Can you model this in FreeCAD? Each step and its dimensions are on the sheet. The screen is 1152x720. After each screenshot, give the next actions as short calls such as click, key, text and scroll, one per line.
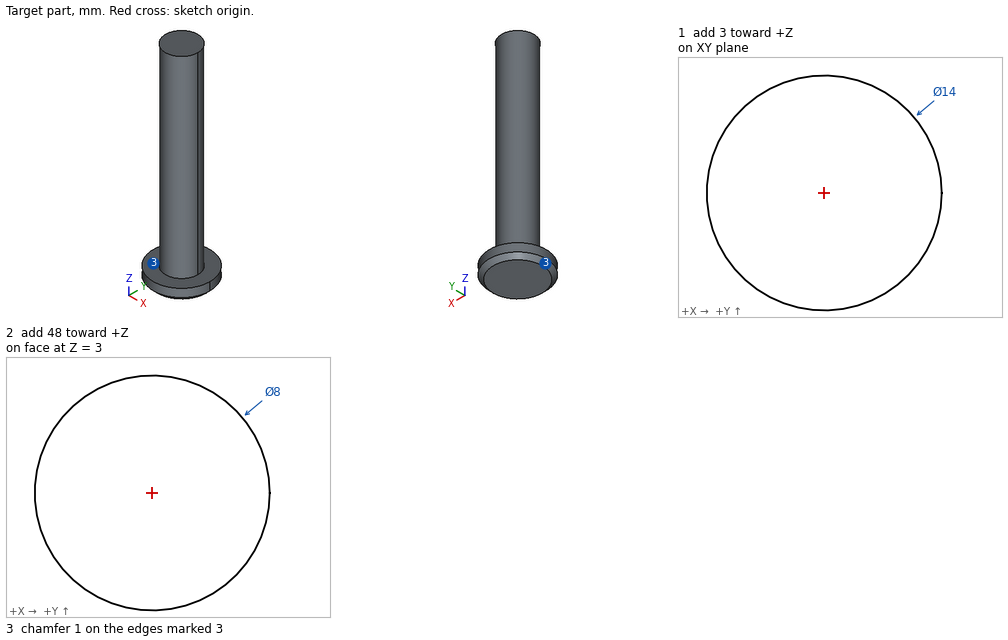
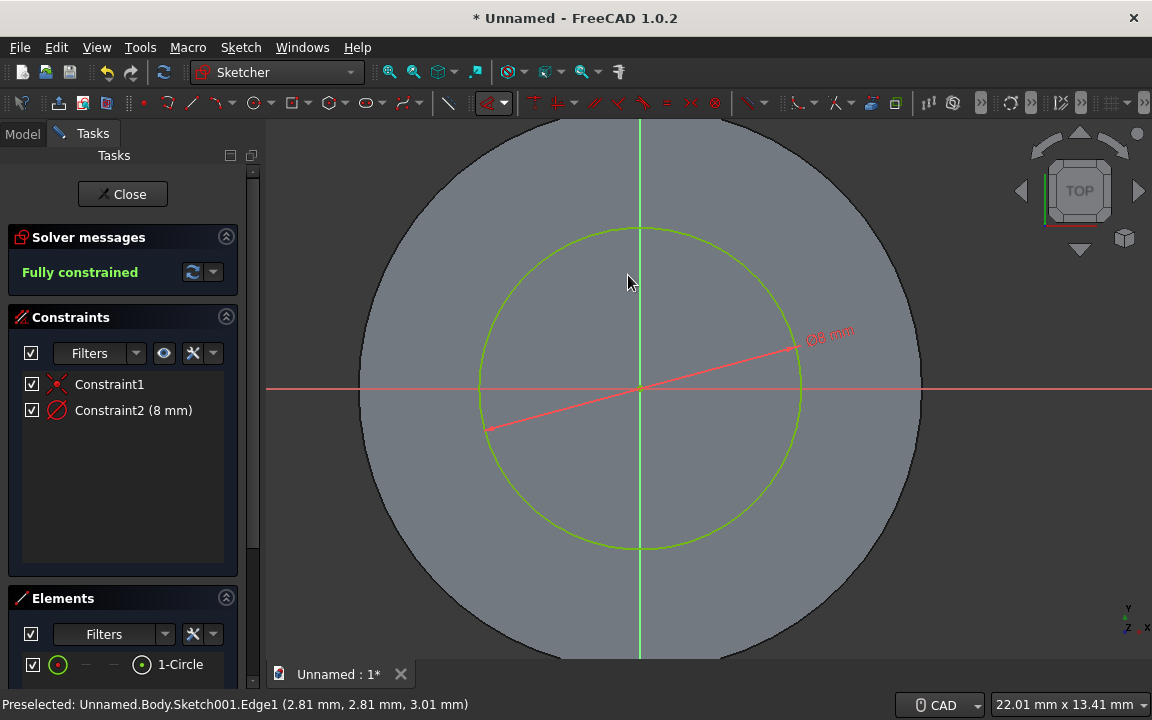
click(123, 194)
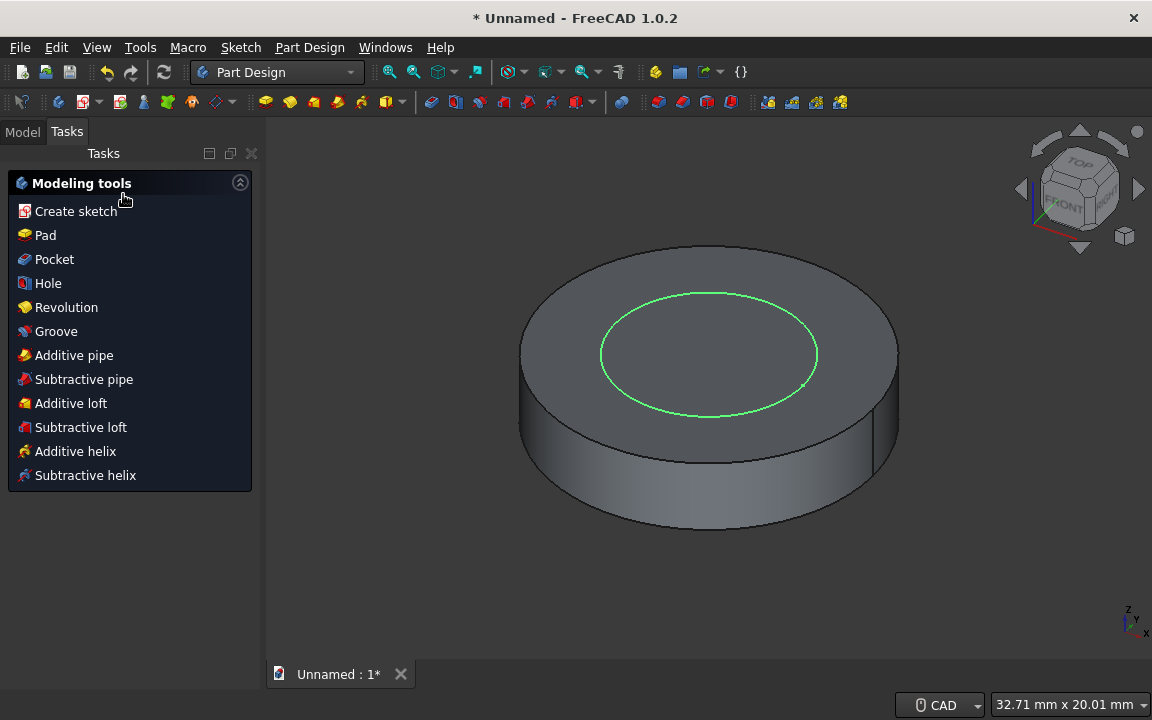
click(266, 102)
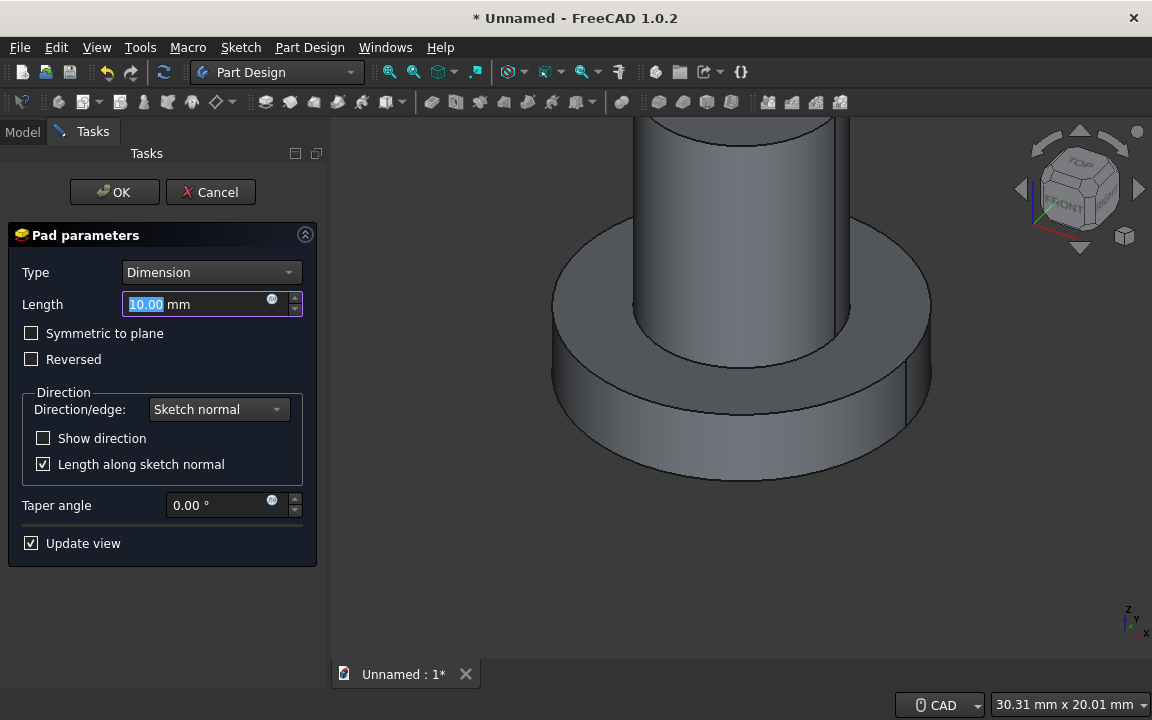
text(48)
key(Tab)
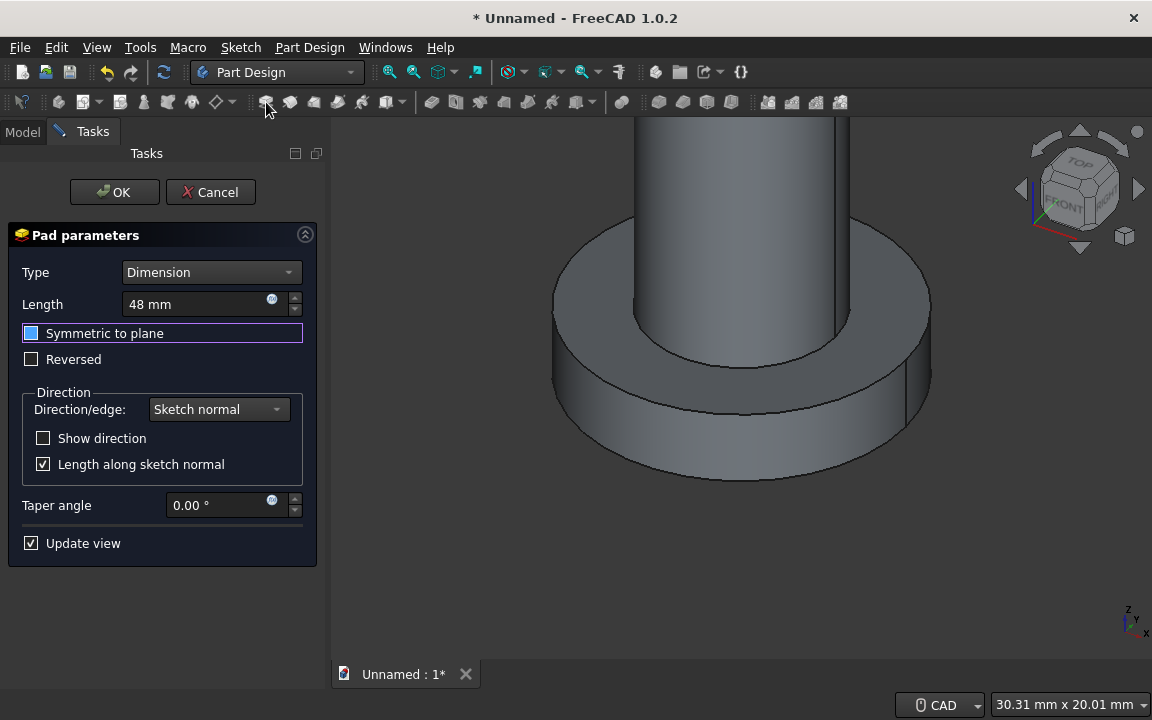
click(115, 192)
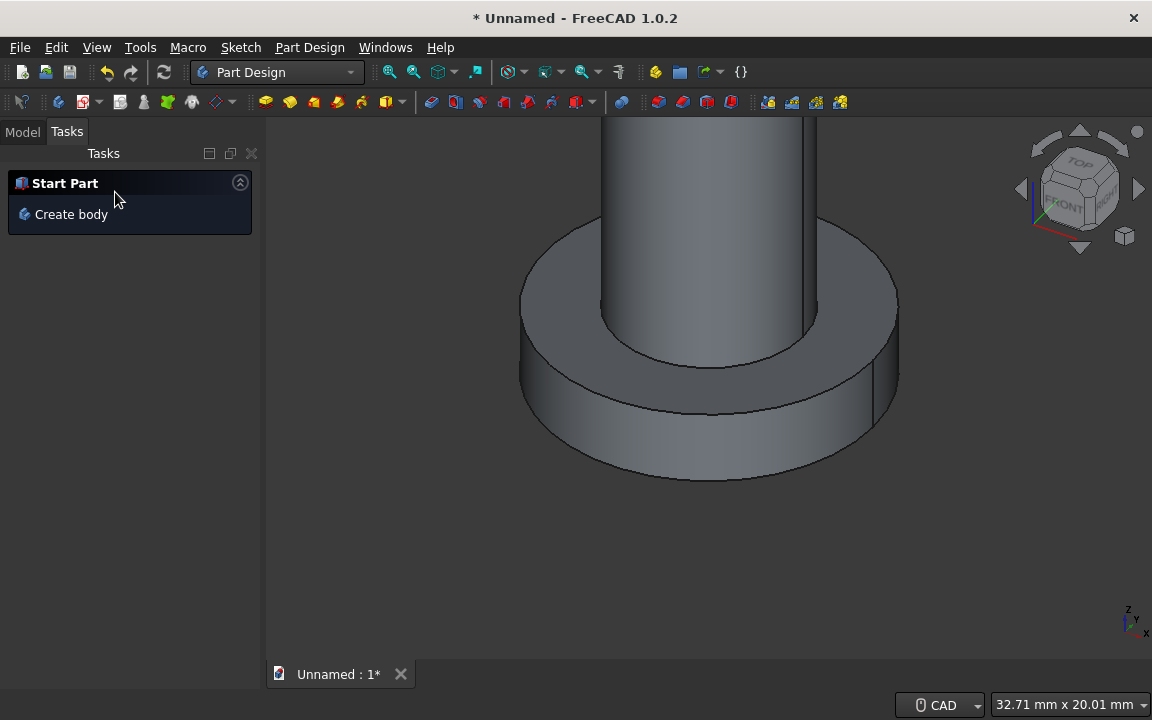
click(390, 72)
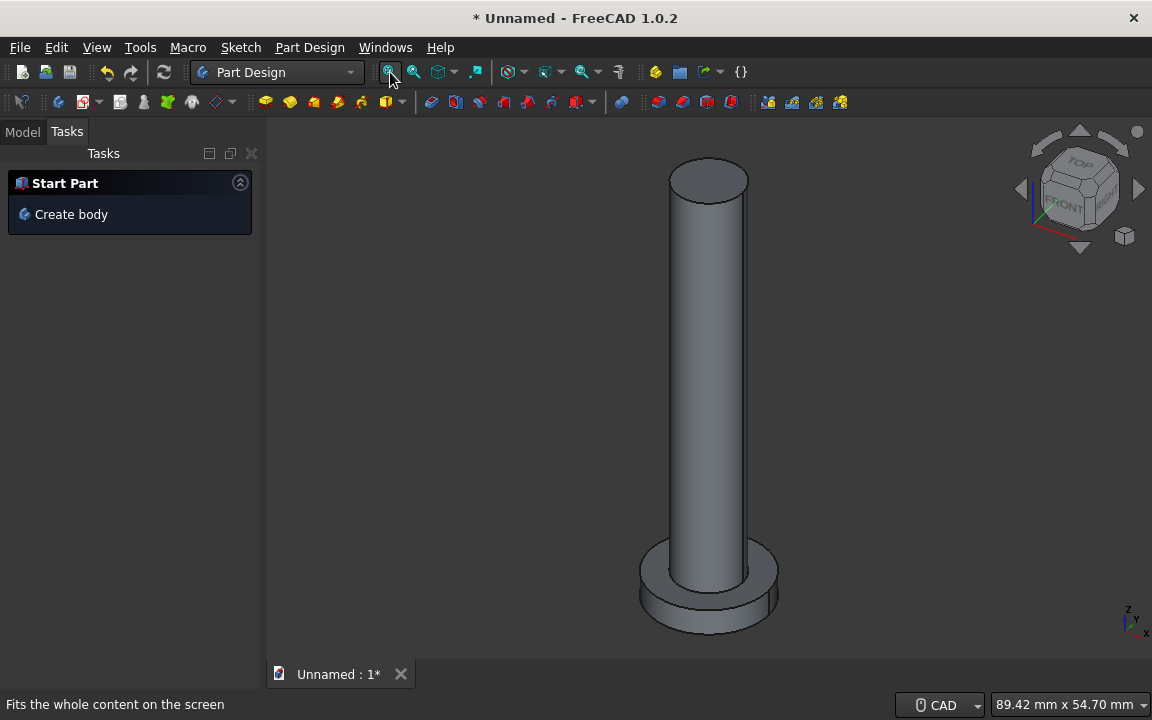
key(0)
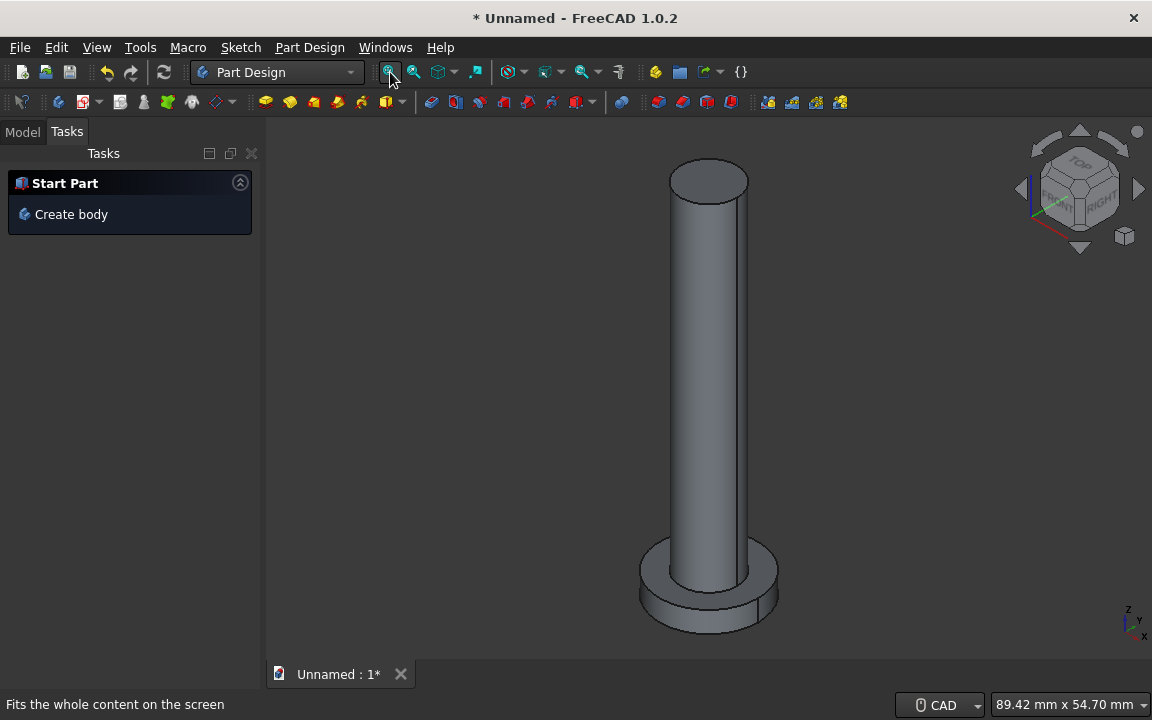
key(2)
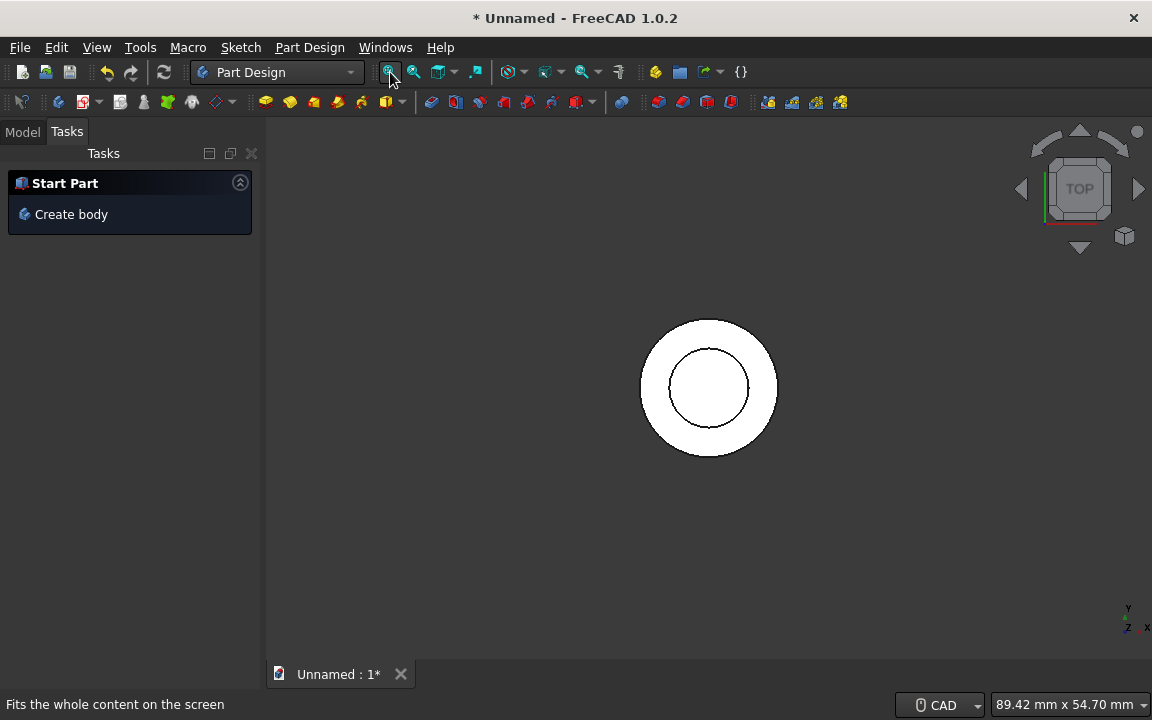
click(390, 72)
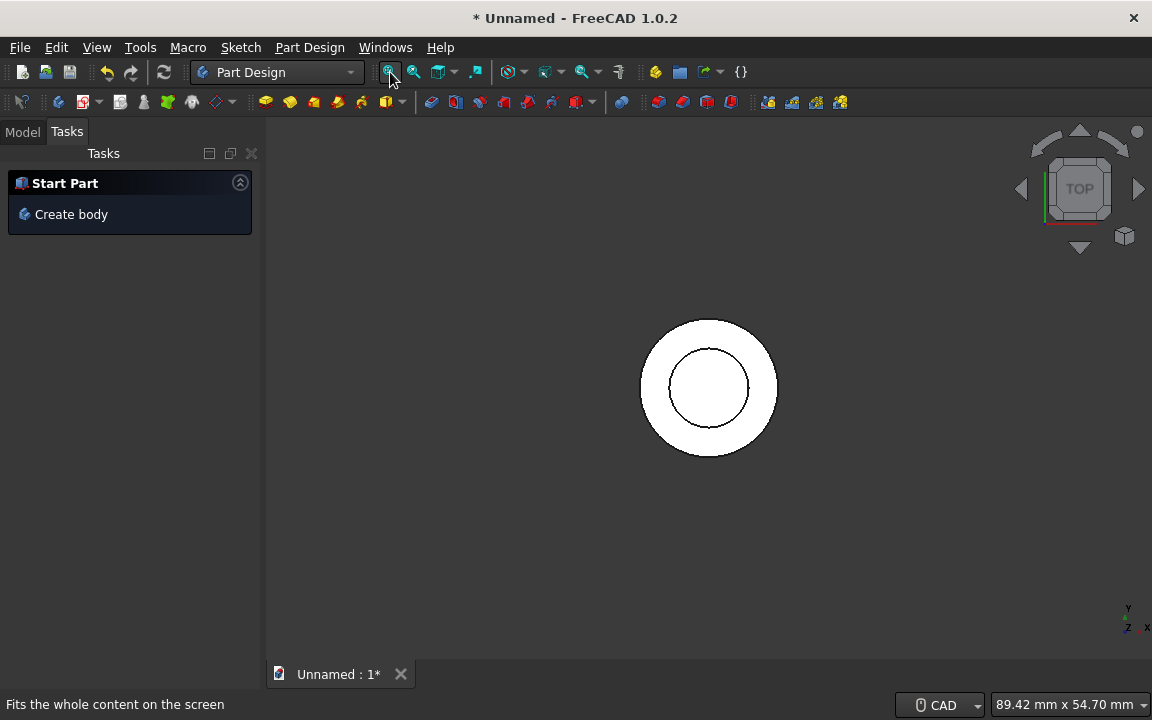
key(1)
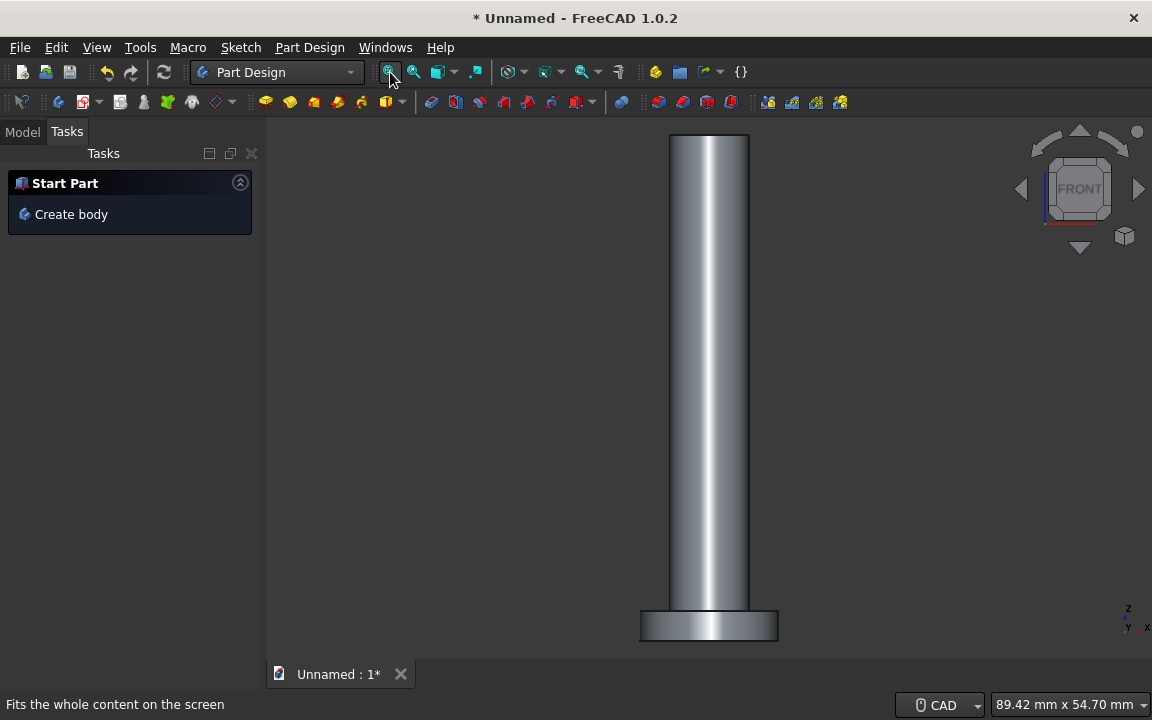
key(3)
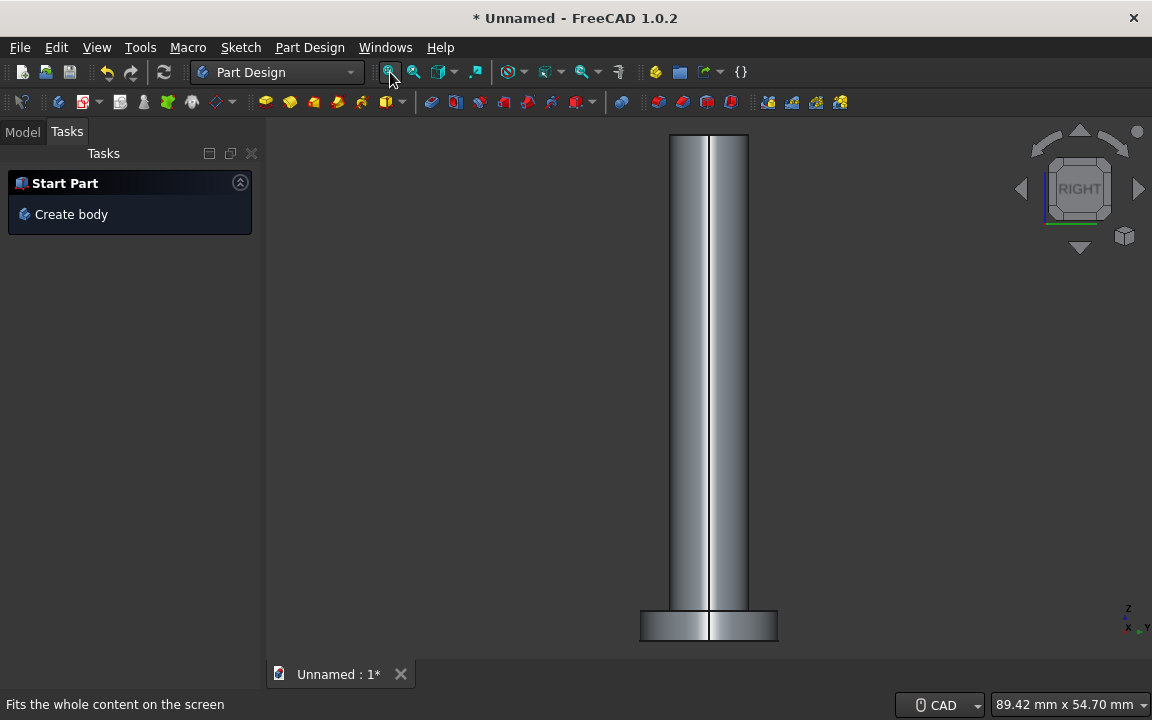
key(5)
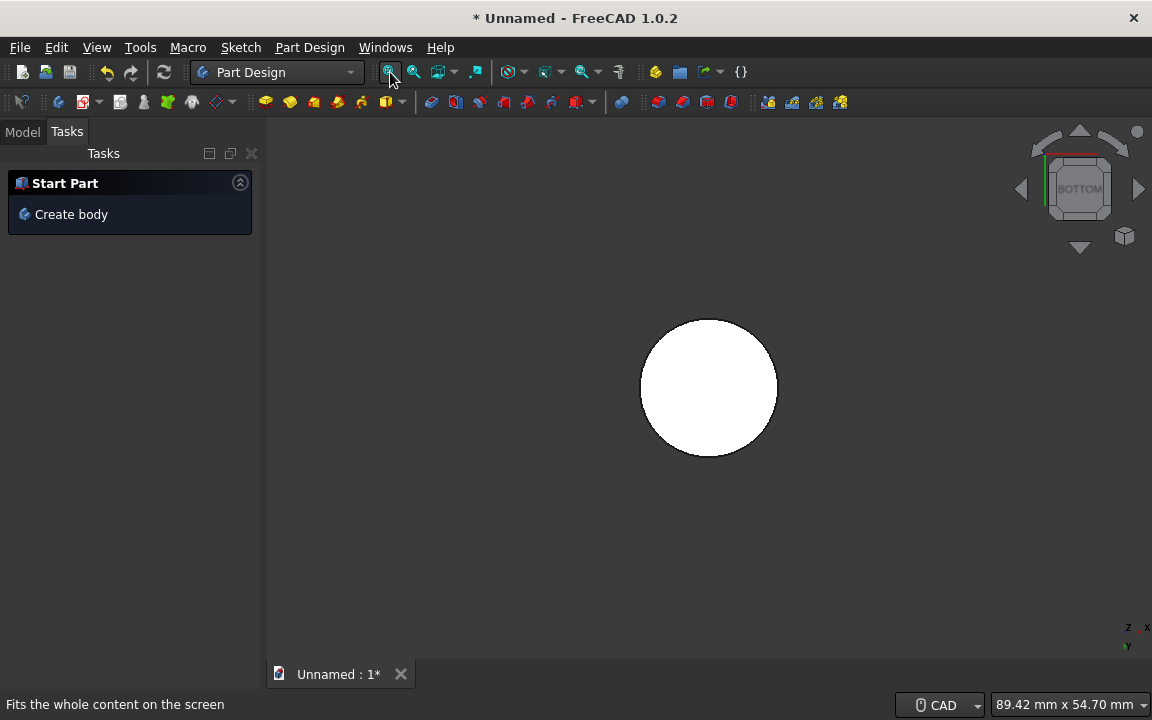
click(390, 72)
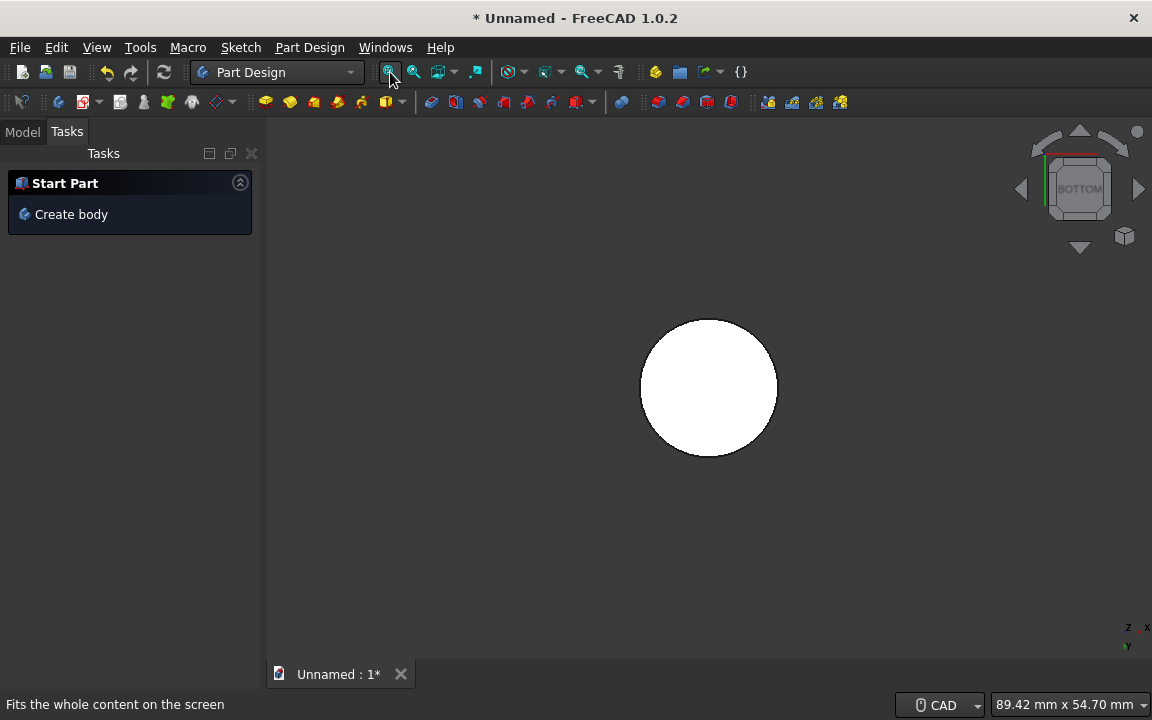
click(653, 428)